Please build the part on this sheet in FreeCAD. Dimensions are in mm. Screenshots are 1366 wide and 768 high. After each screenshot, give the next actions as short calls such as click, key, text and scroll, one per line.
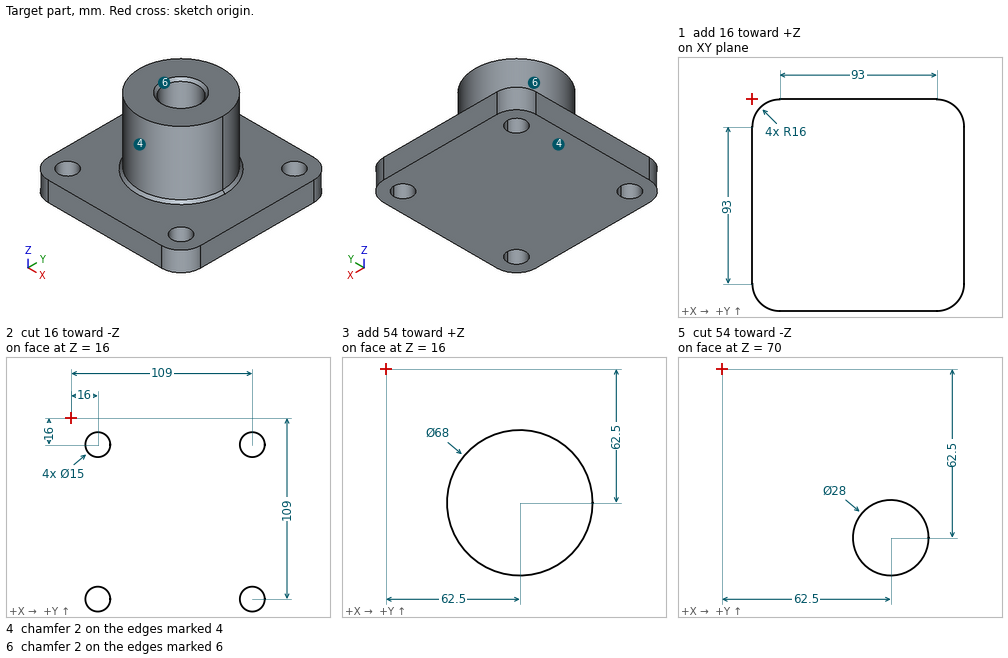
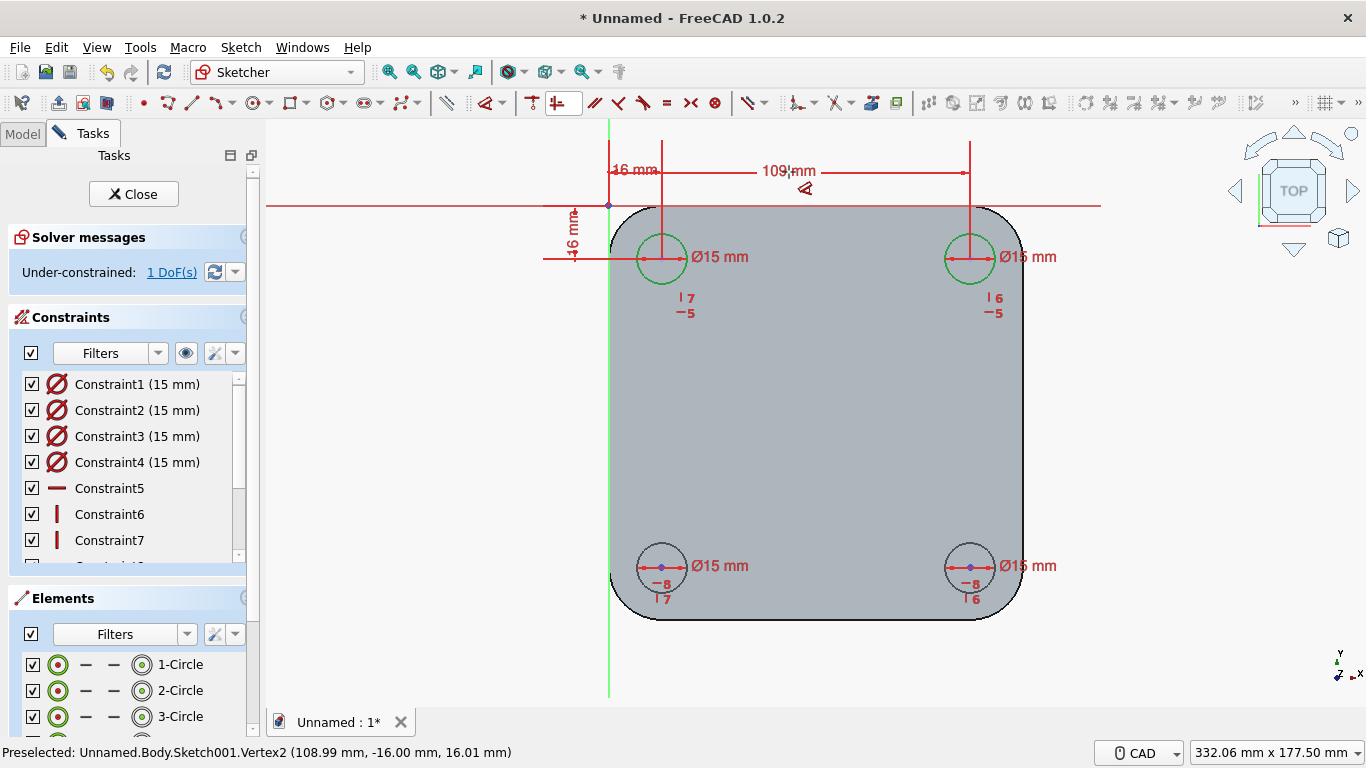
click(970, 568)
click(575, 387)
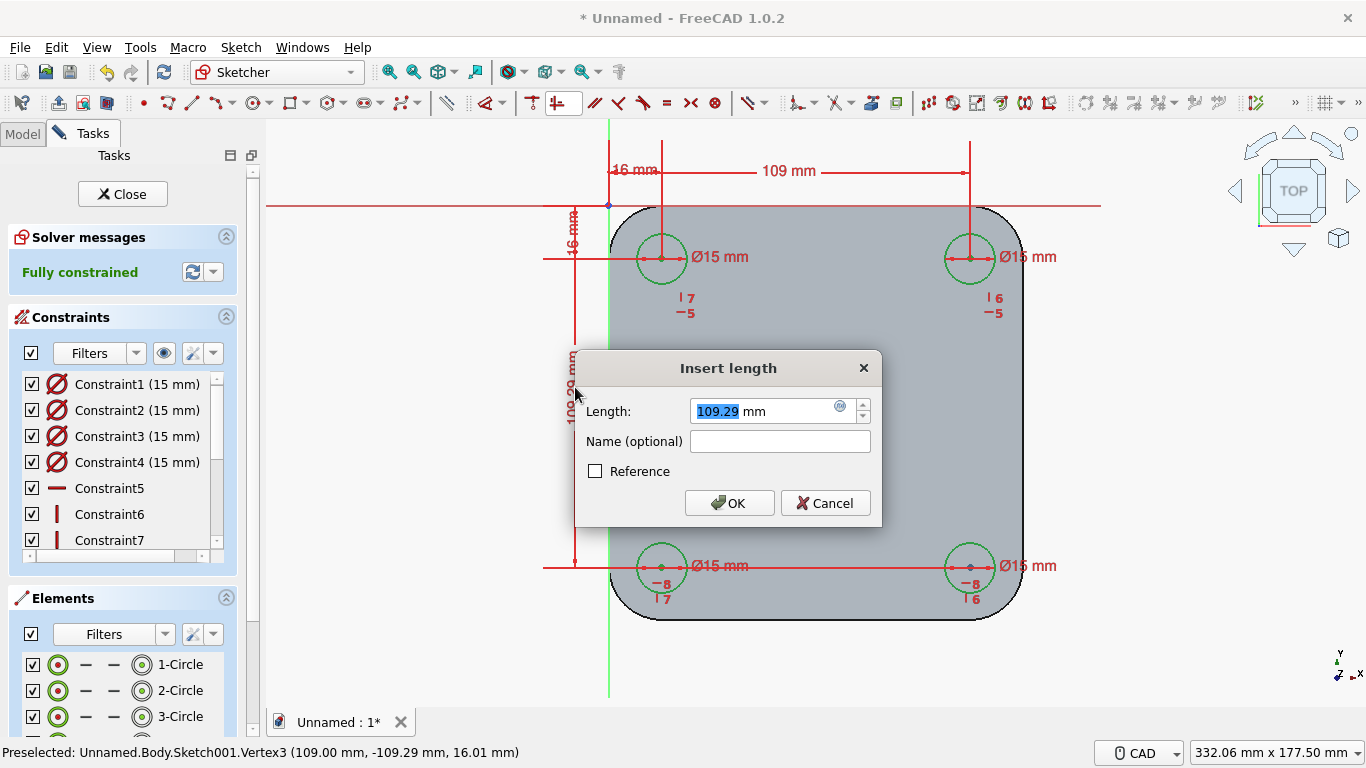
text(109)
key(Return)
key(Escape)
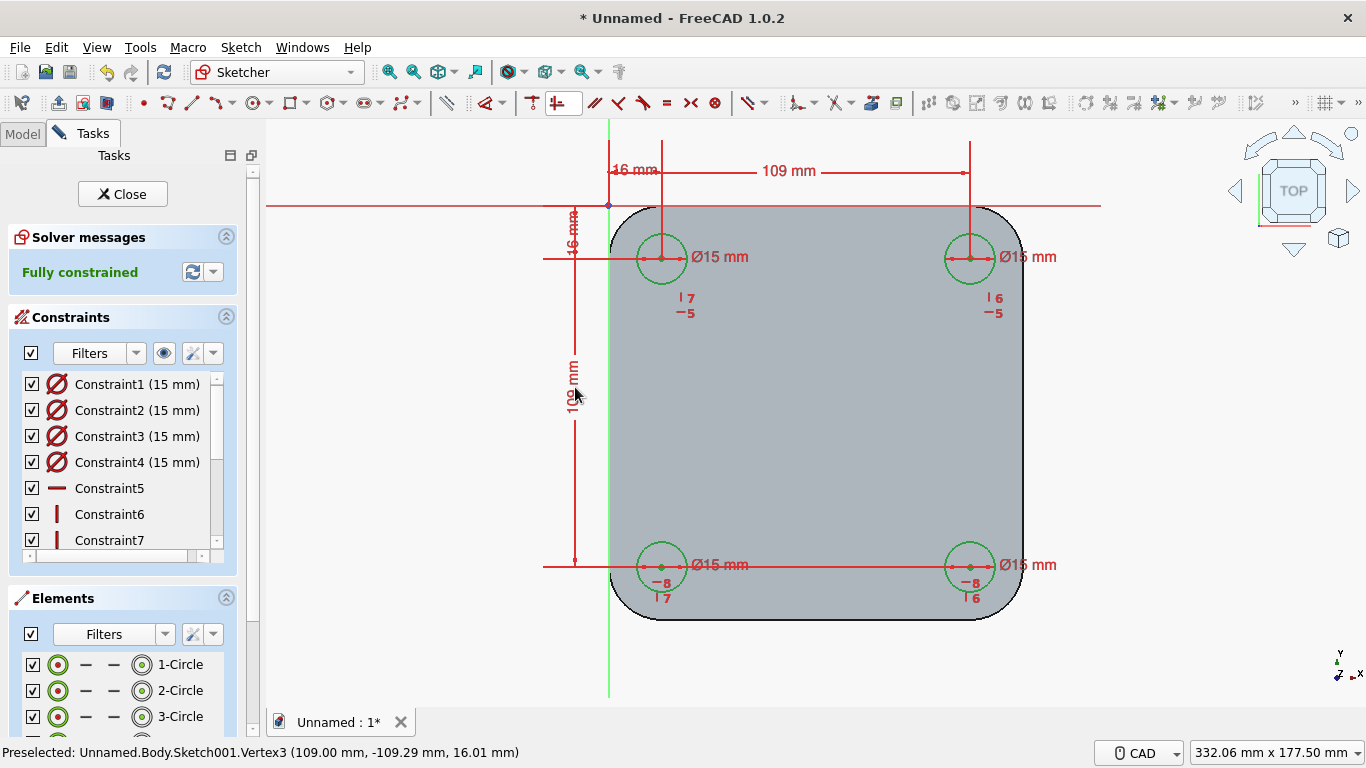
click(123, 194)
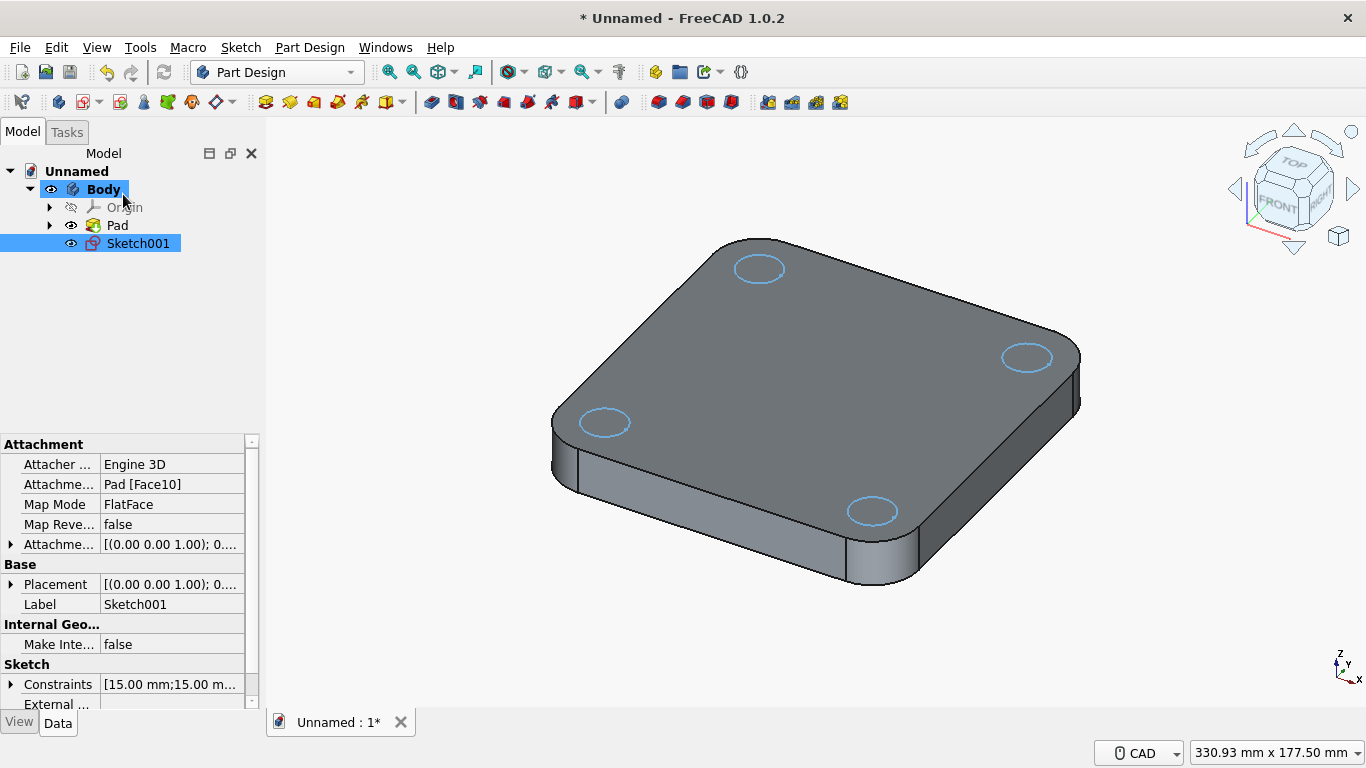
click(432, 102)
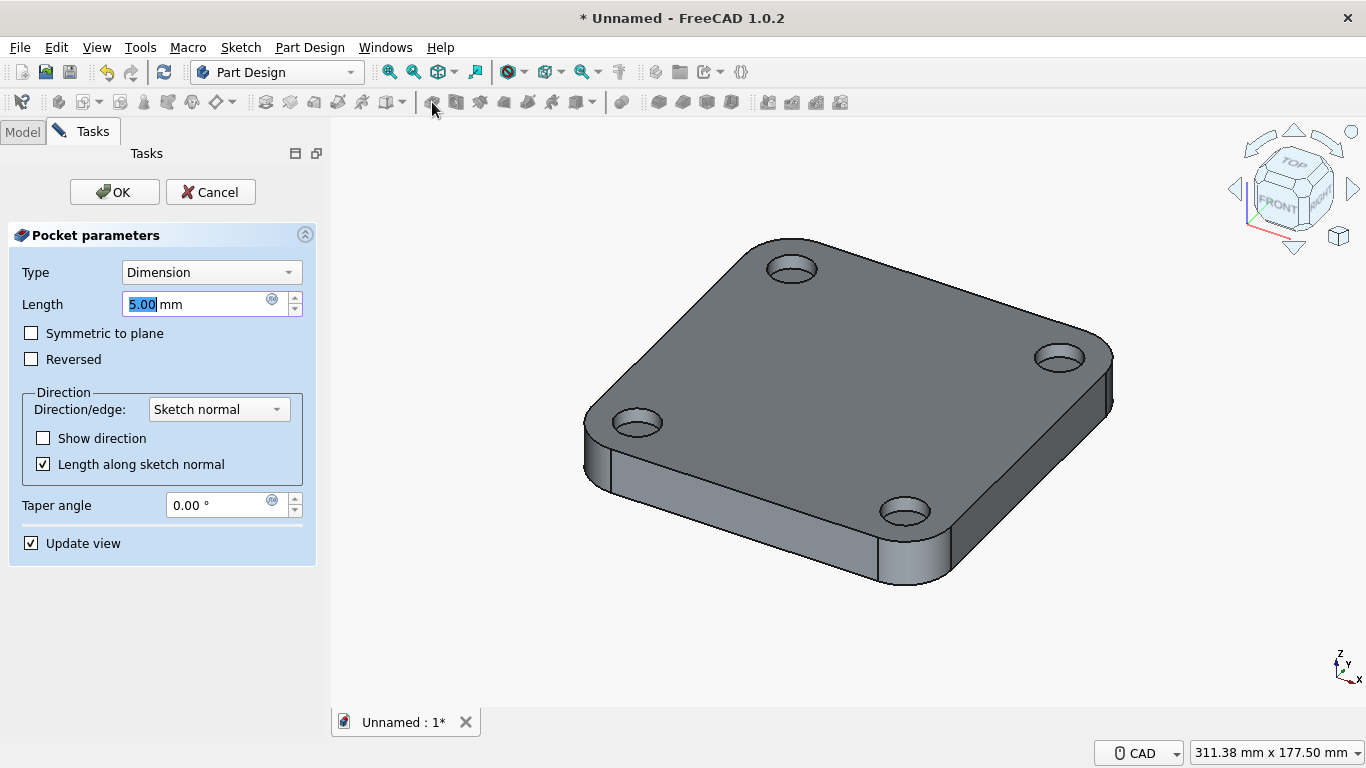
text(16)
key(Tab)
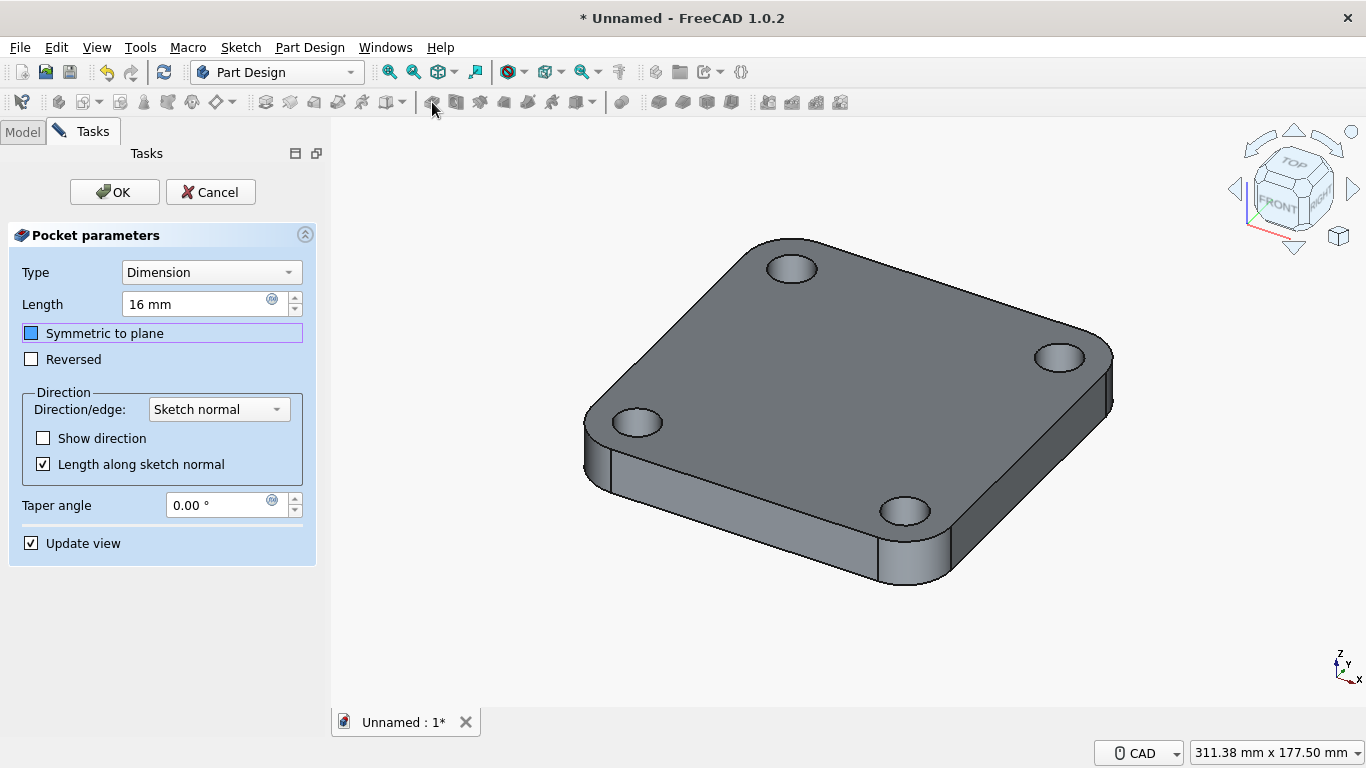
click(115, 192)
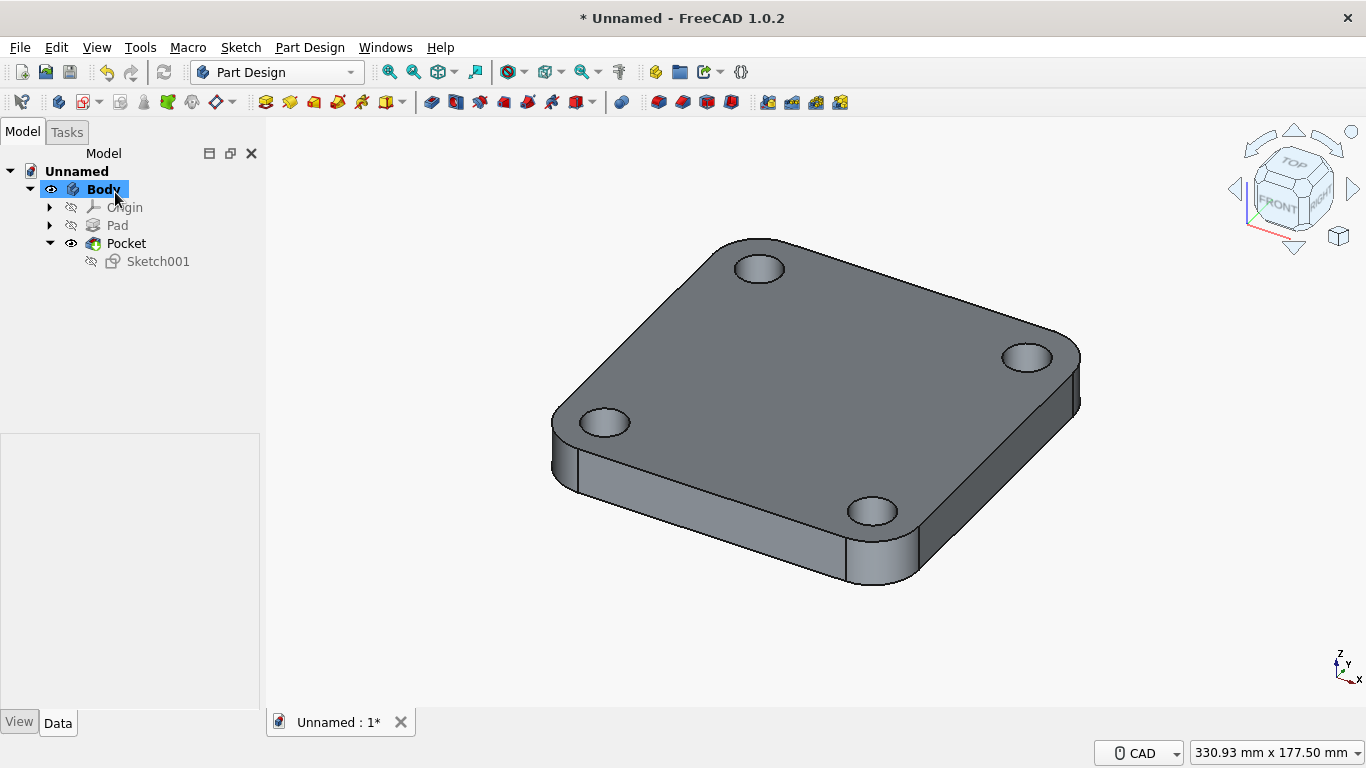
click(816, 389)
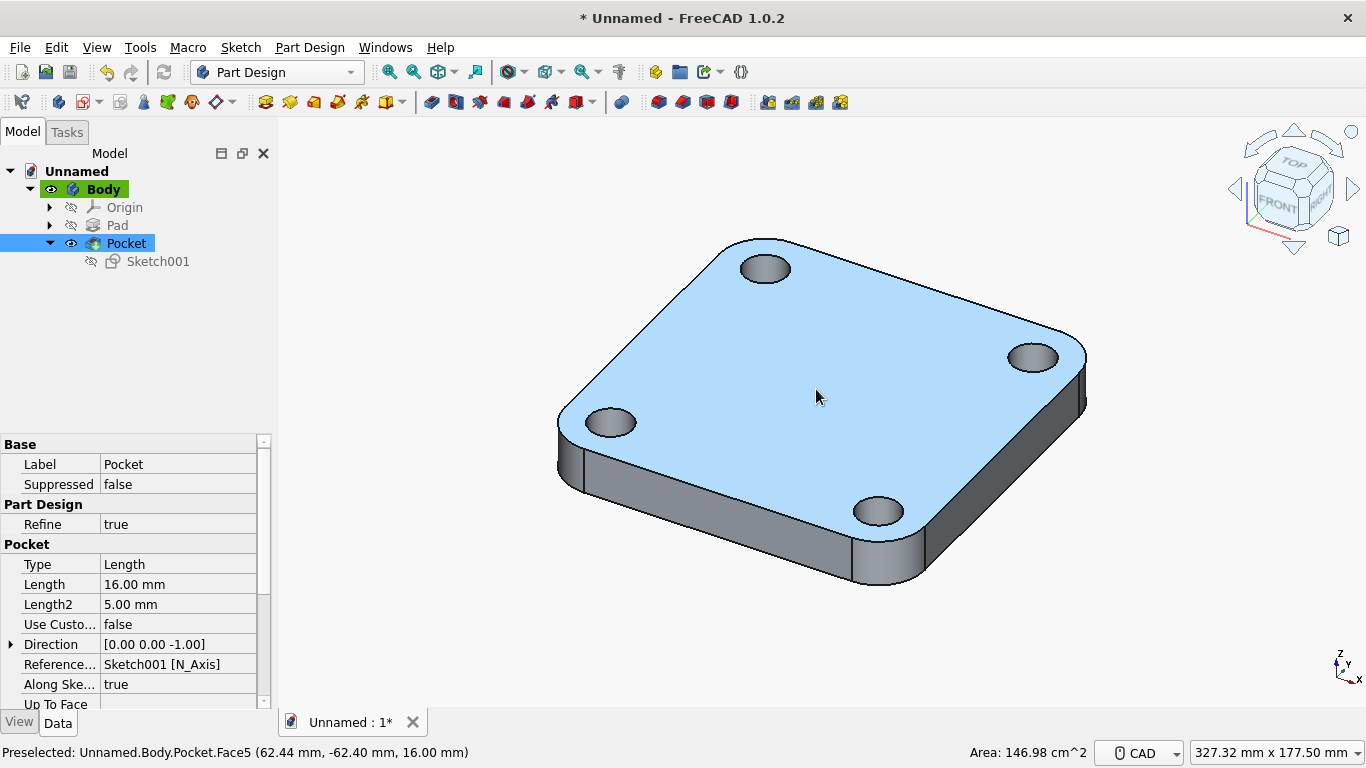
click(84, 102)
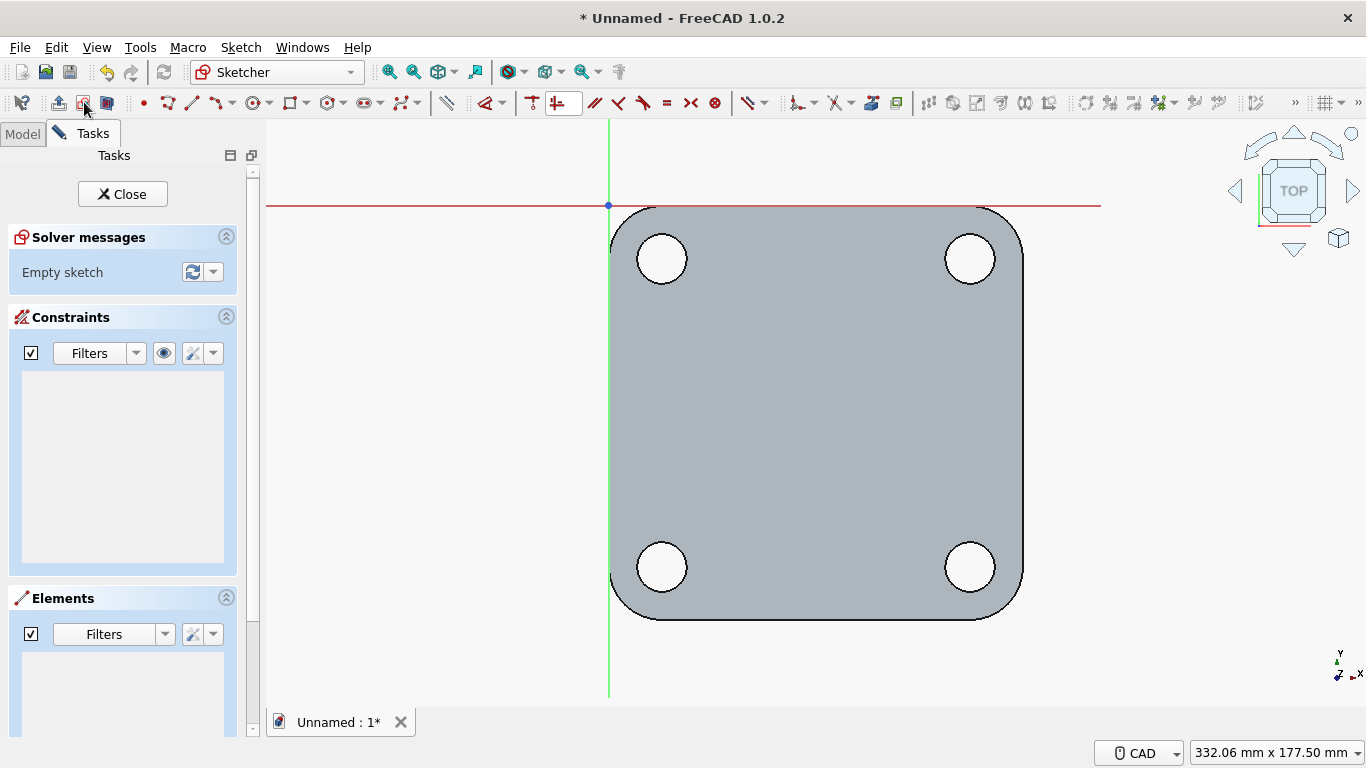
click(254, 104)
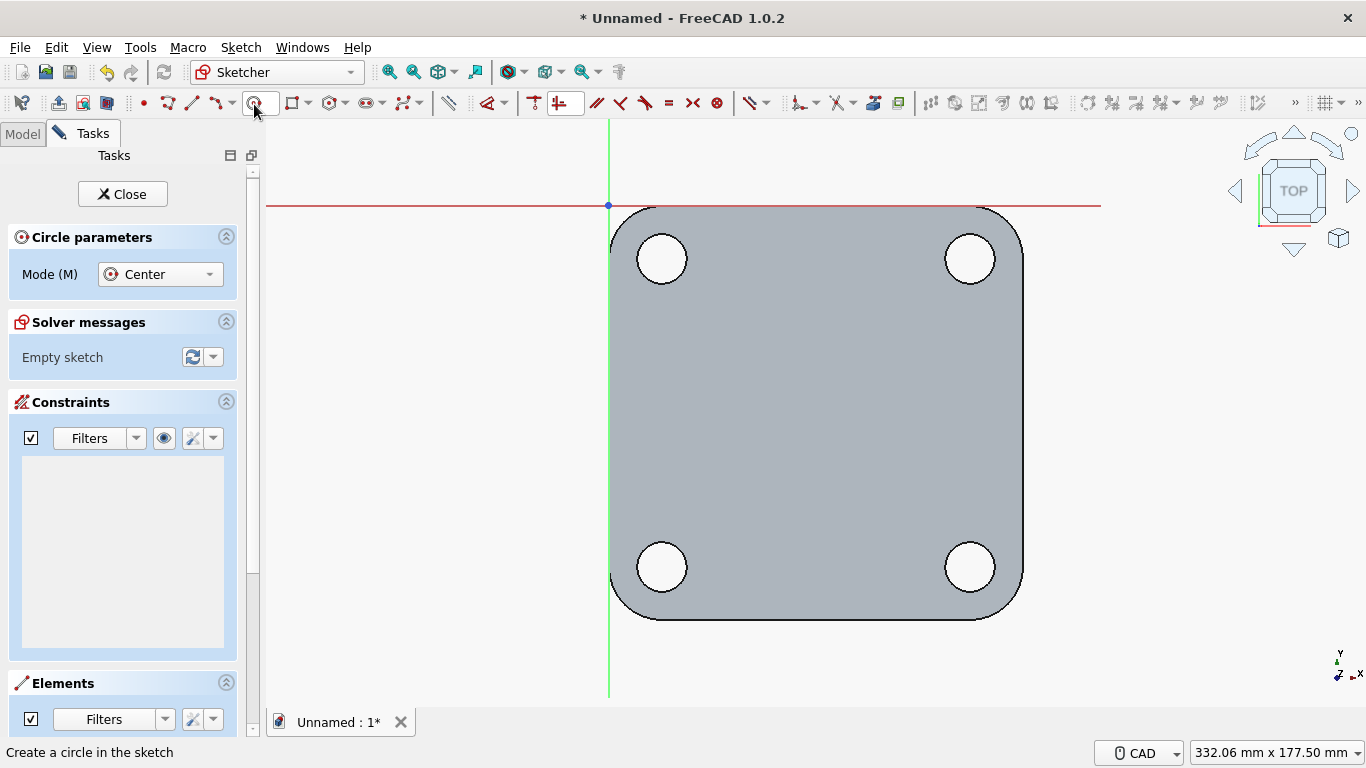
click(816, 413)
move(896, 333)